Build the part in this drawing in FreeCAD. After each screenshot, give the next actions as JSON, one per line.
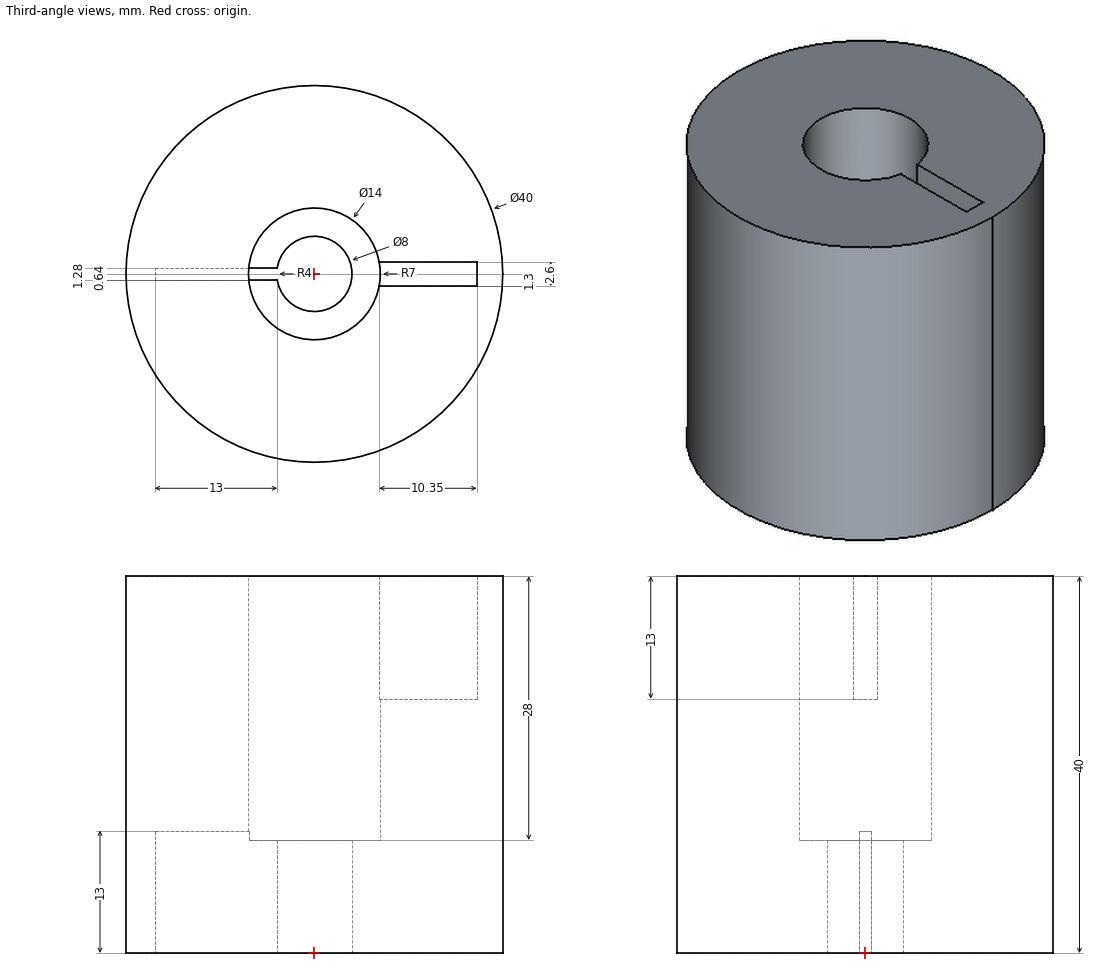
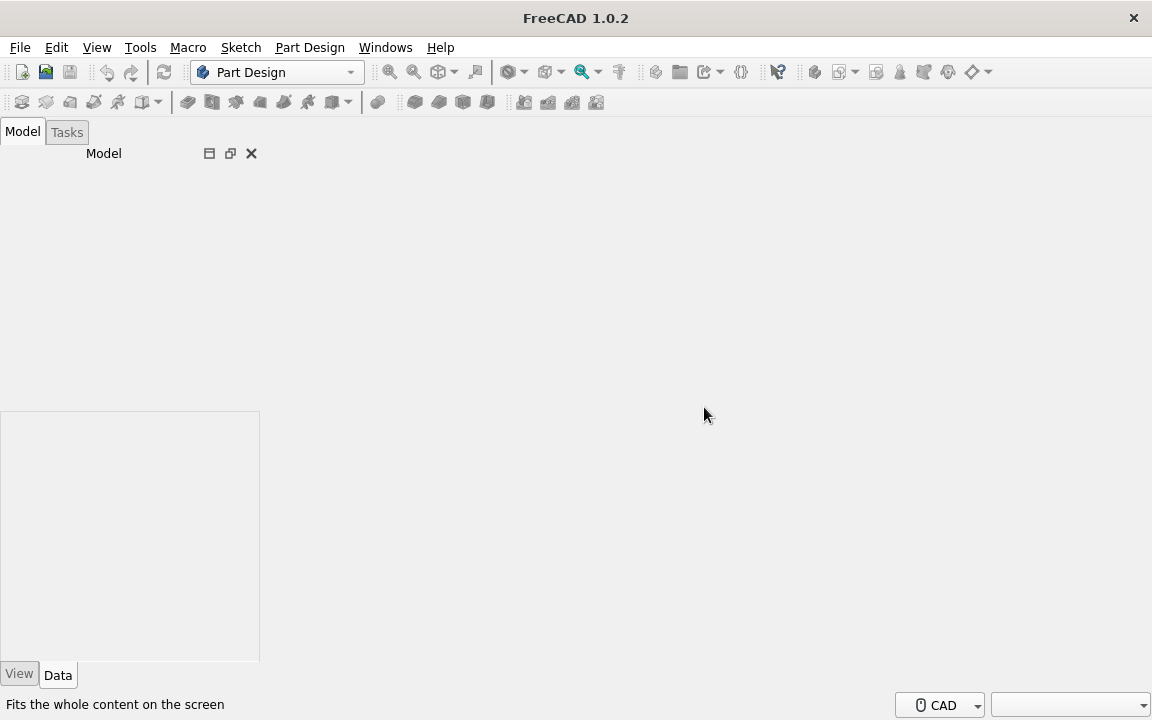
{"action": "left_click", "coordinate": [22, 72]}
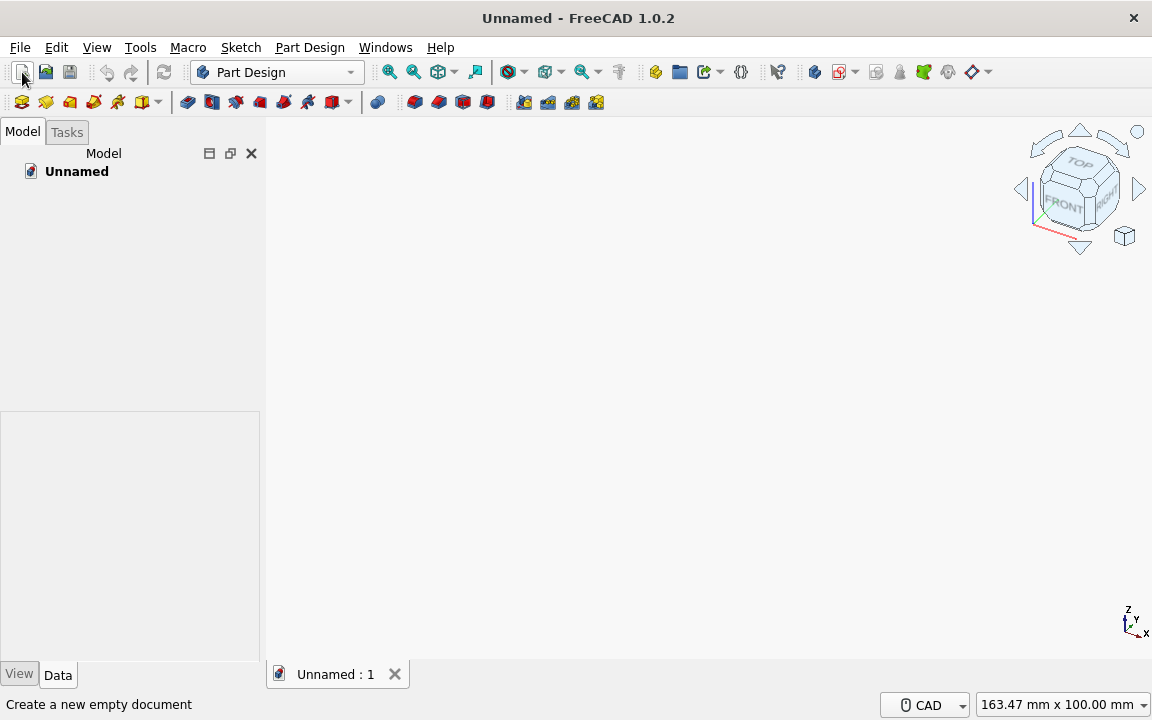
{"action": "left_click", "coordinate": [840, 72]}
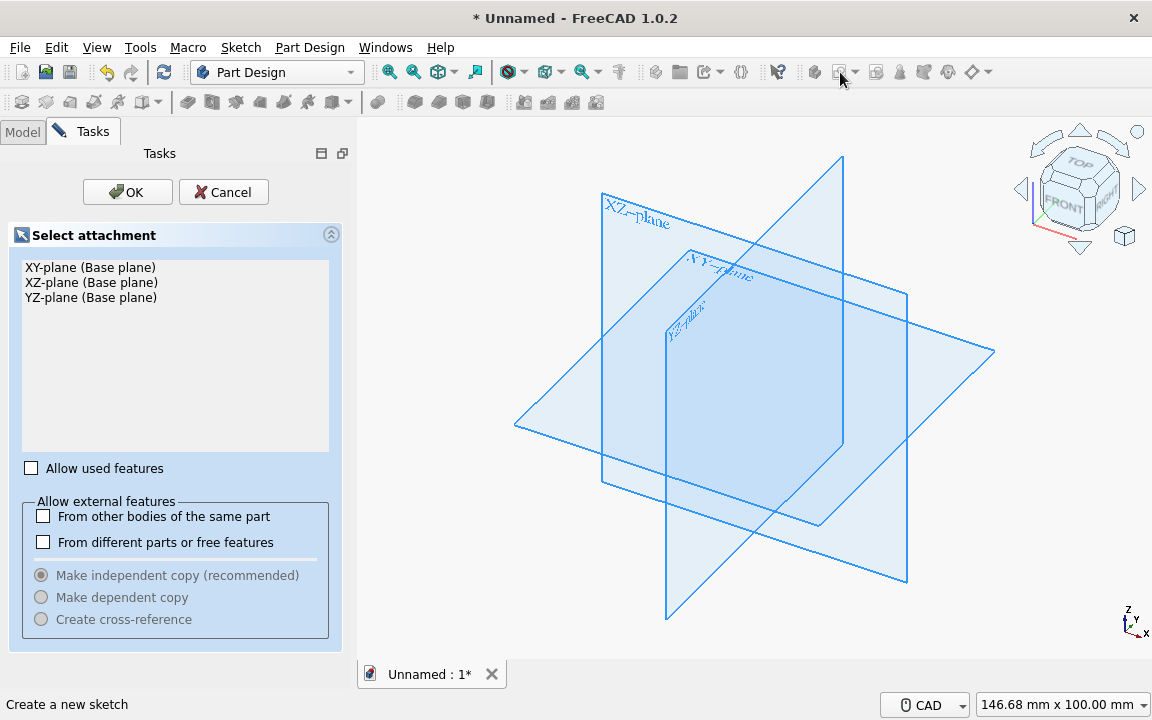
{"action": "left_click", "coordinate": [82, 268]}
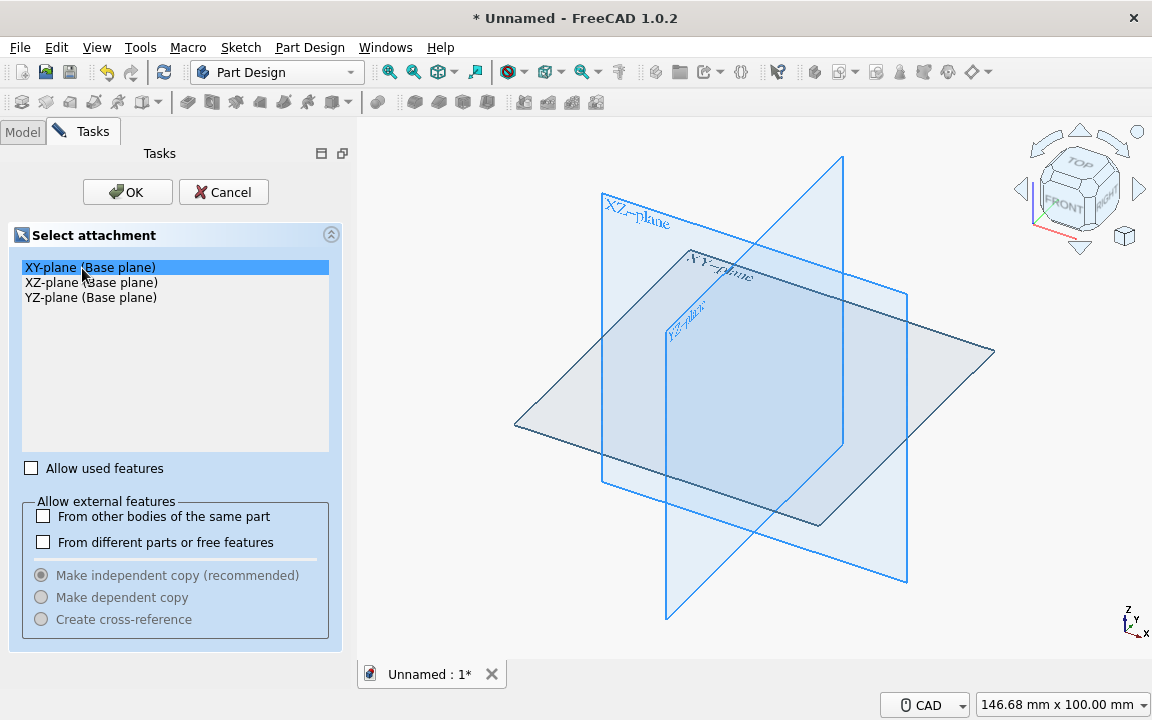
{"action": "left_click", "coordinate": [128, 192]}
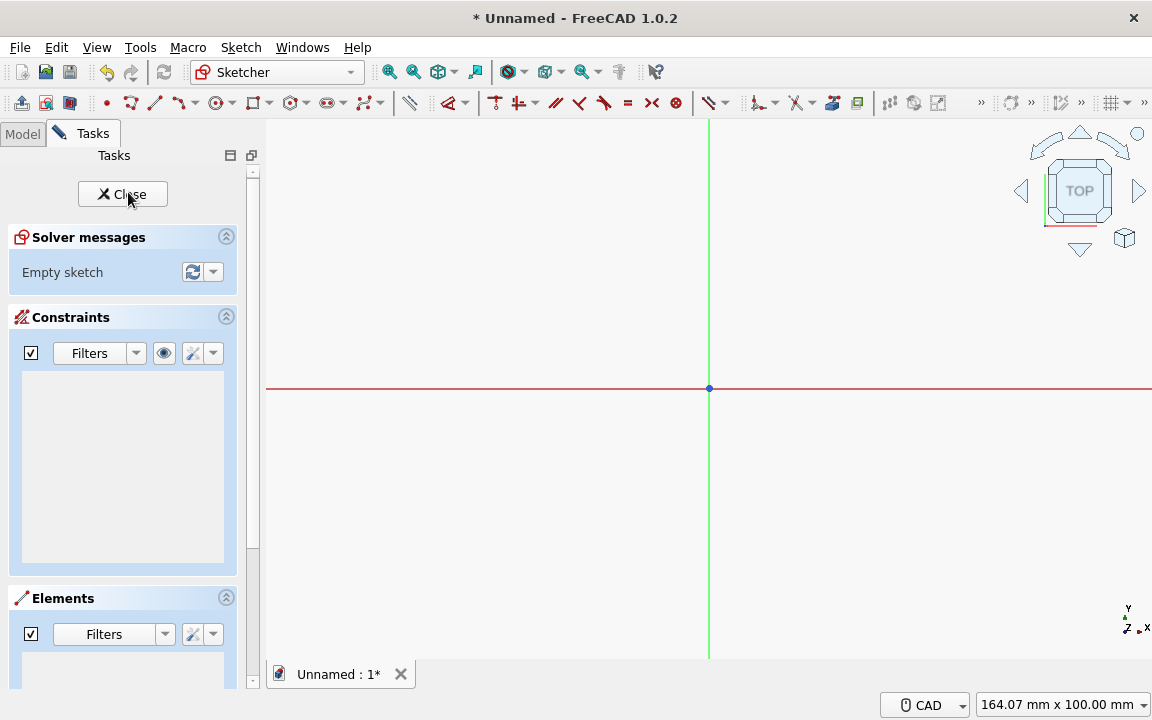
{"action": "scroll", "coordinate": [848, 389], "scroll_direction": "up", "scroll_amount": 2}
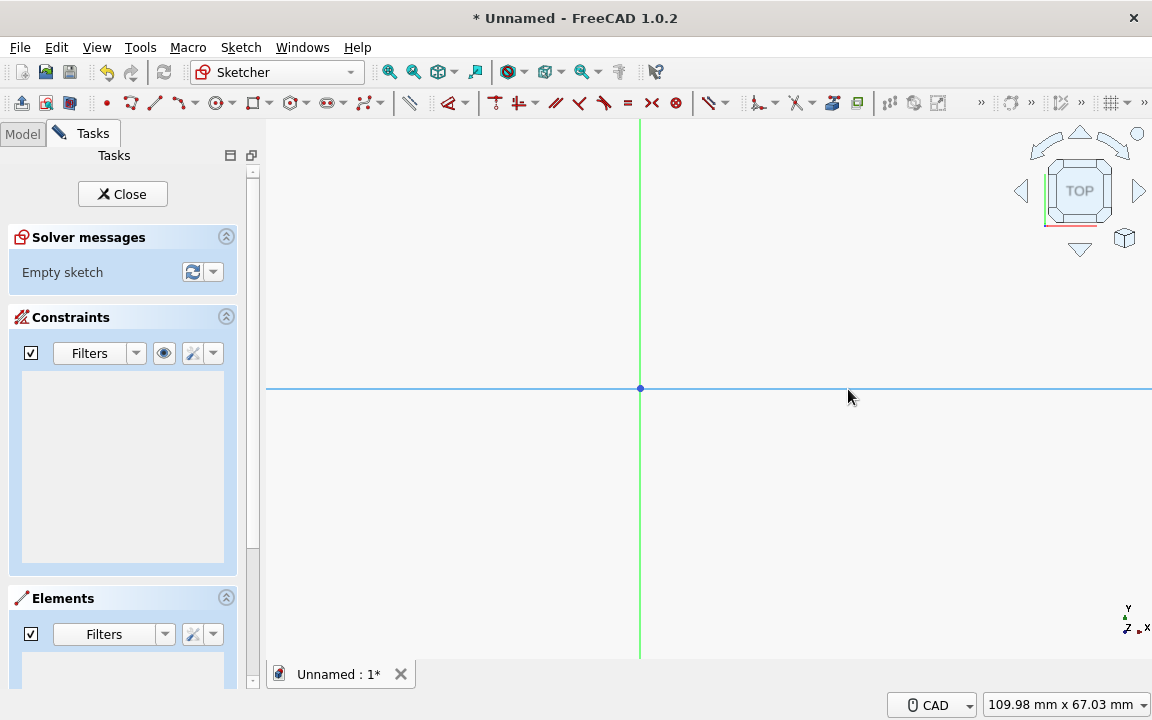
{"action": "left_click", "coordinate": [216, 104]}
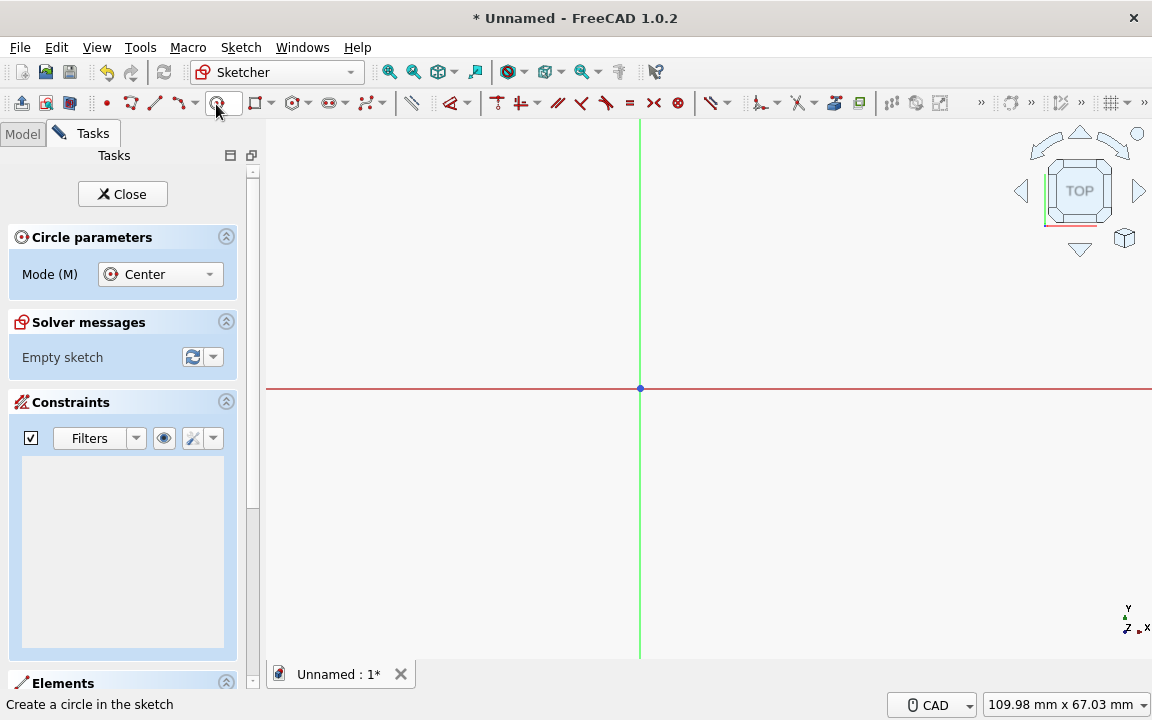
{"action": "left_click", "coordinate": [640, 389]}
{"action": "left_click", "coordinate": [754, 275]}
{"action": "key", "text": "Escape"}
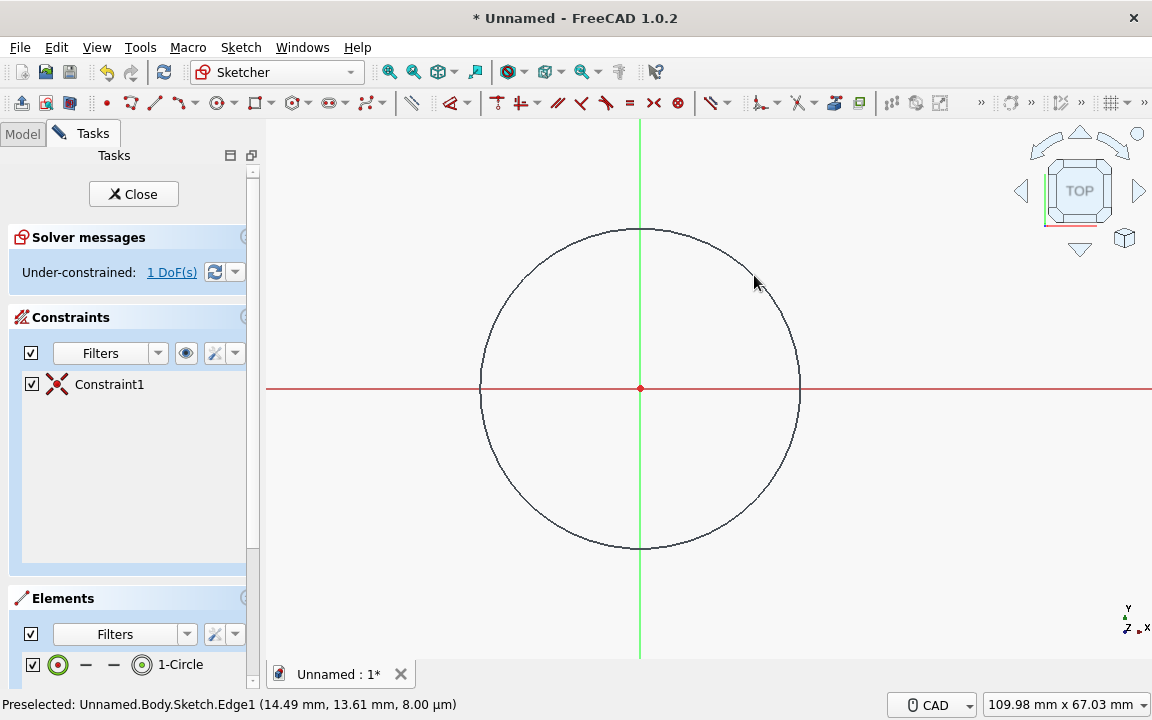
{"action": "key", "text": "d"}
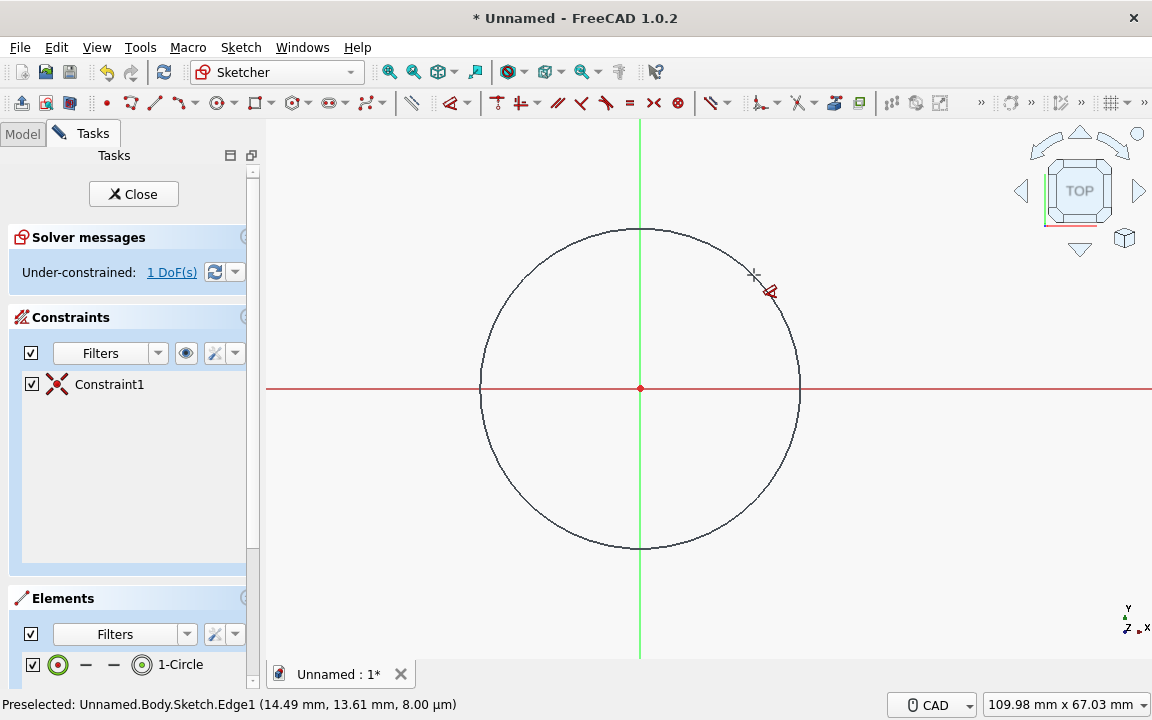
{"action": "left_click", "coordinate": [753, 275]}
{"action": "left_click", "coordinate": [776, 252]}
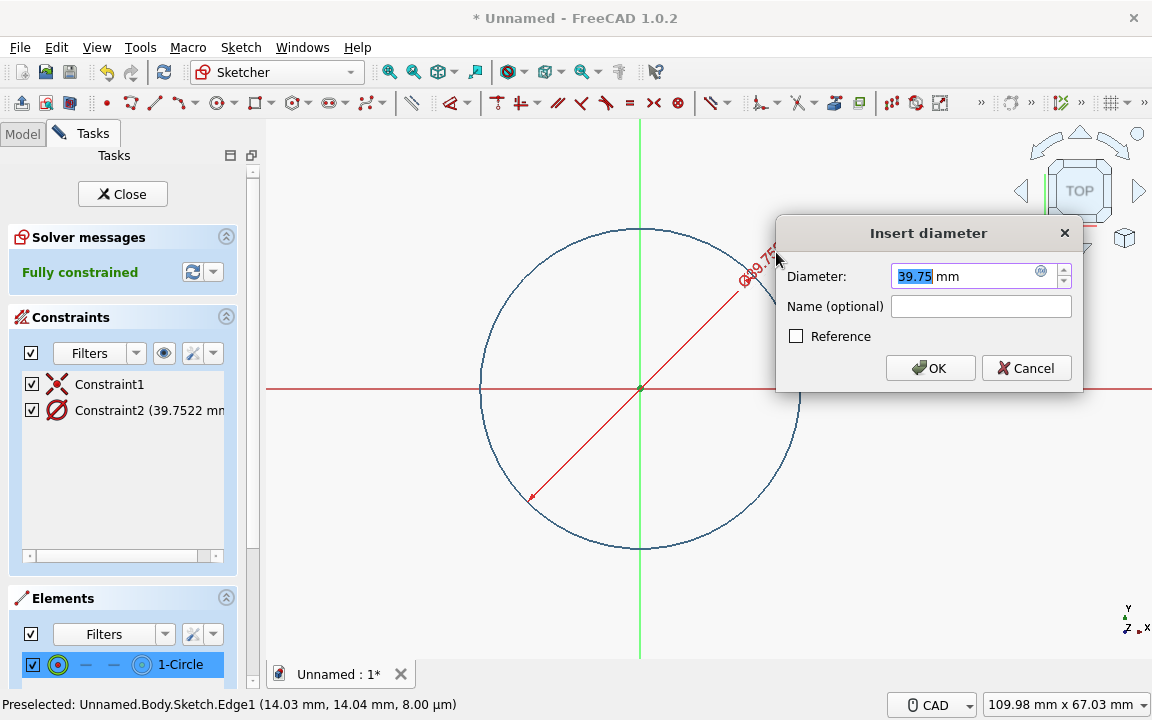
{"action": "type", "text": "40"}
{"action": "key", "text": "Return"}
{"action": "key", "text": "Escape"}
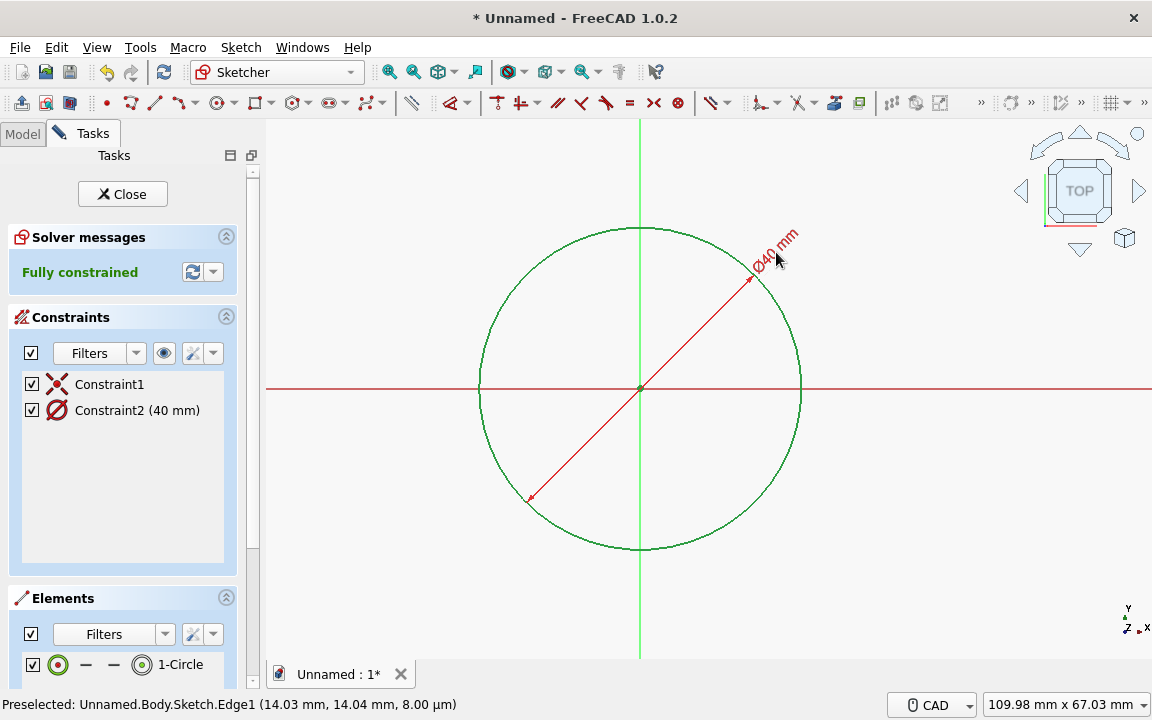
{"action": "left_click", "coordinate": [123, 194]}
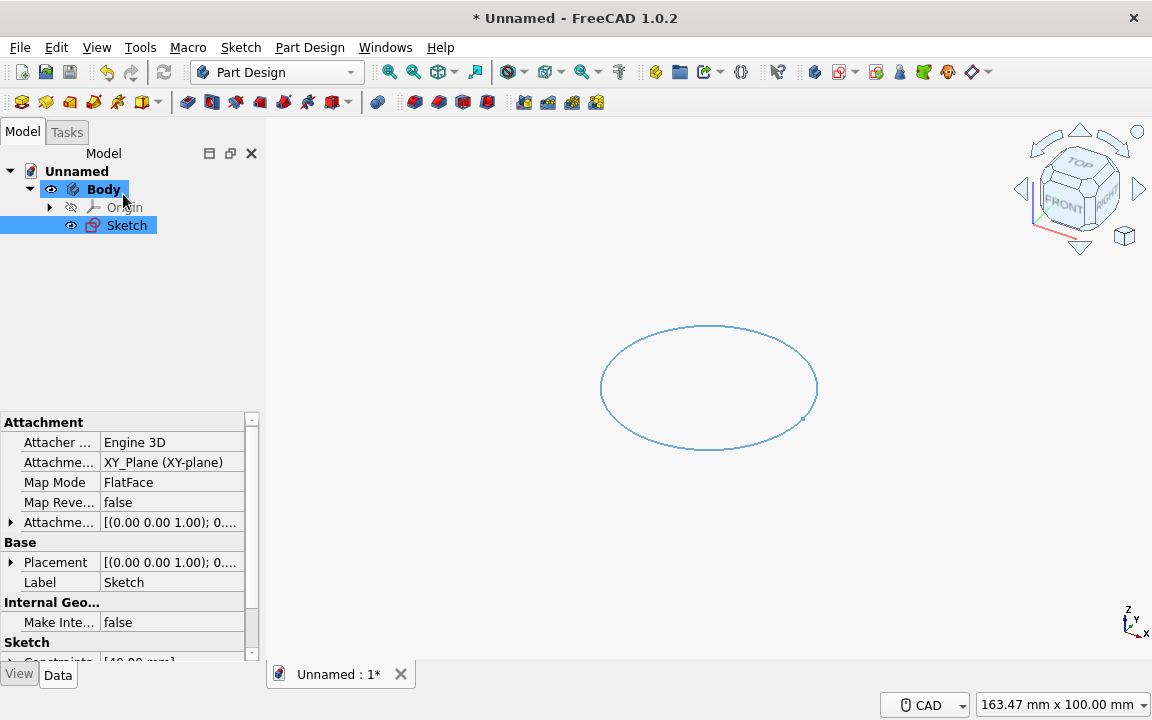
{"action": "left_click", "coordinate": [22, 102]}